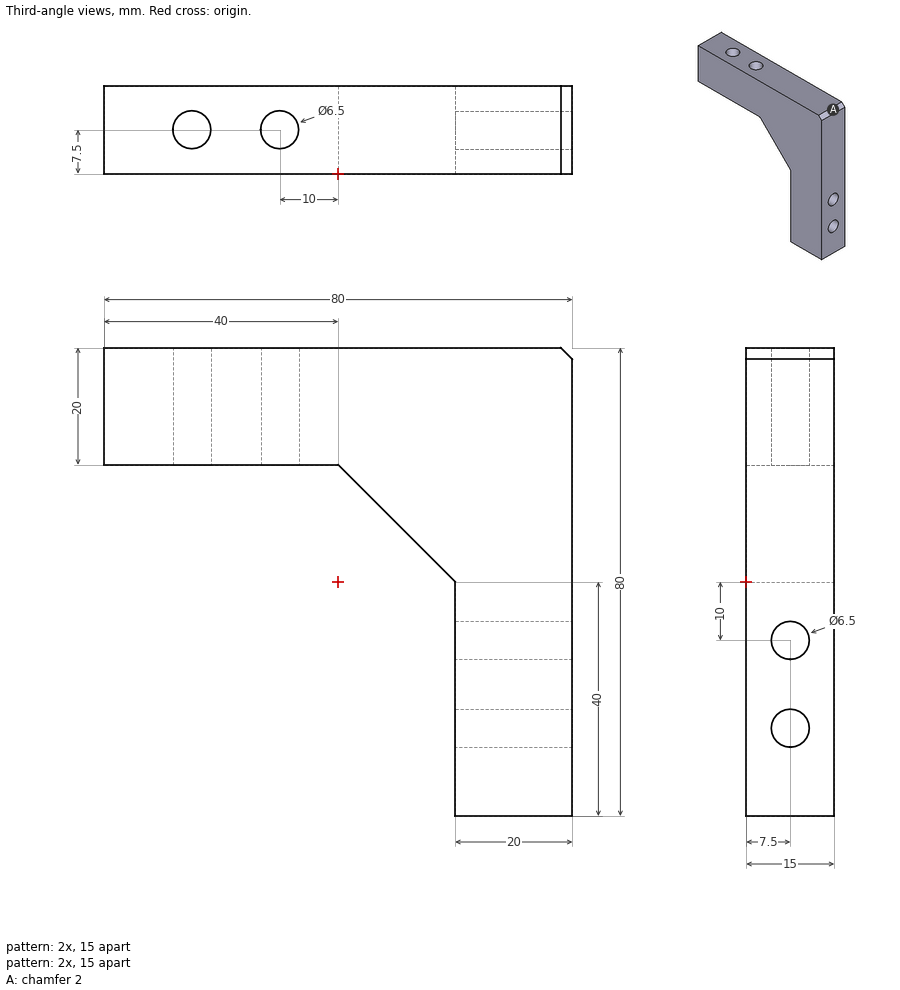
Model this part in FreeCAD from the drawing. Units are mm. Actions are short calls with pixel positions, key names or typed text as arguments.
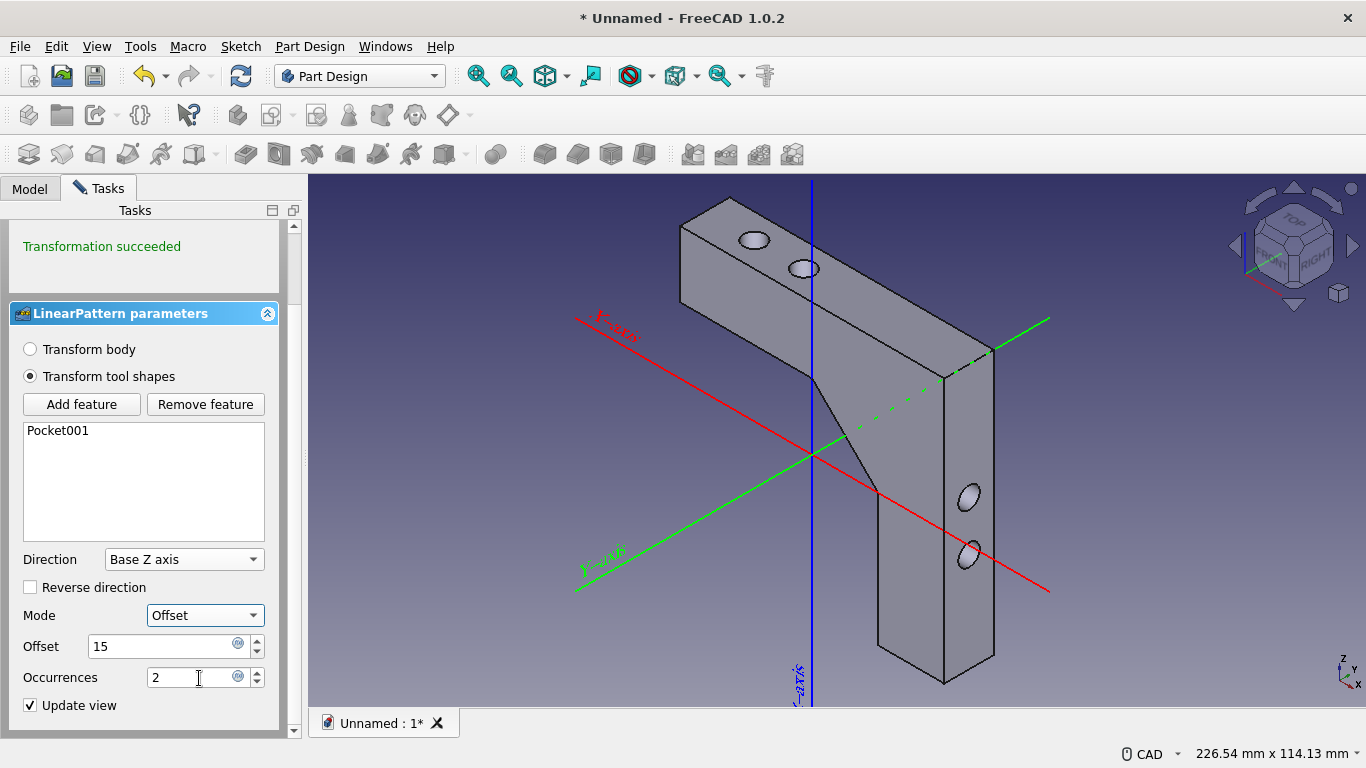
click(31, 587)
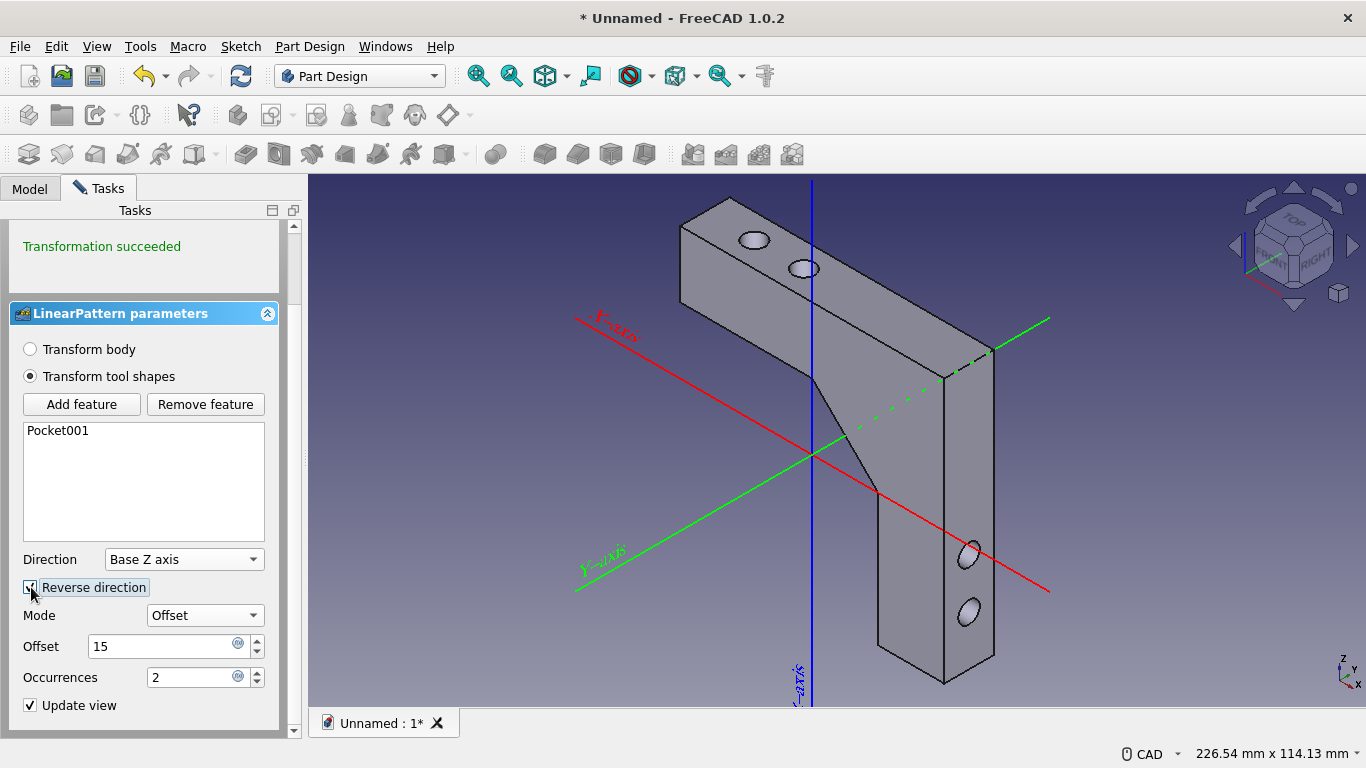
scroll(294, 479, up, 3)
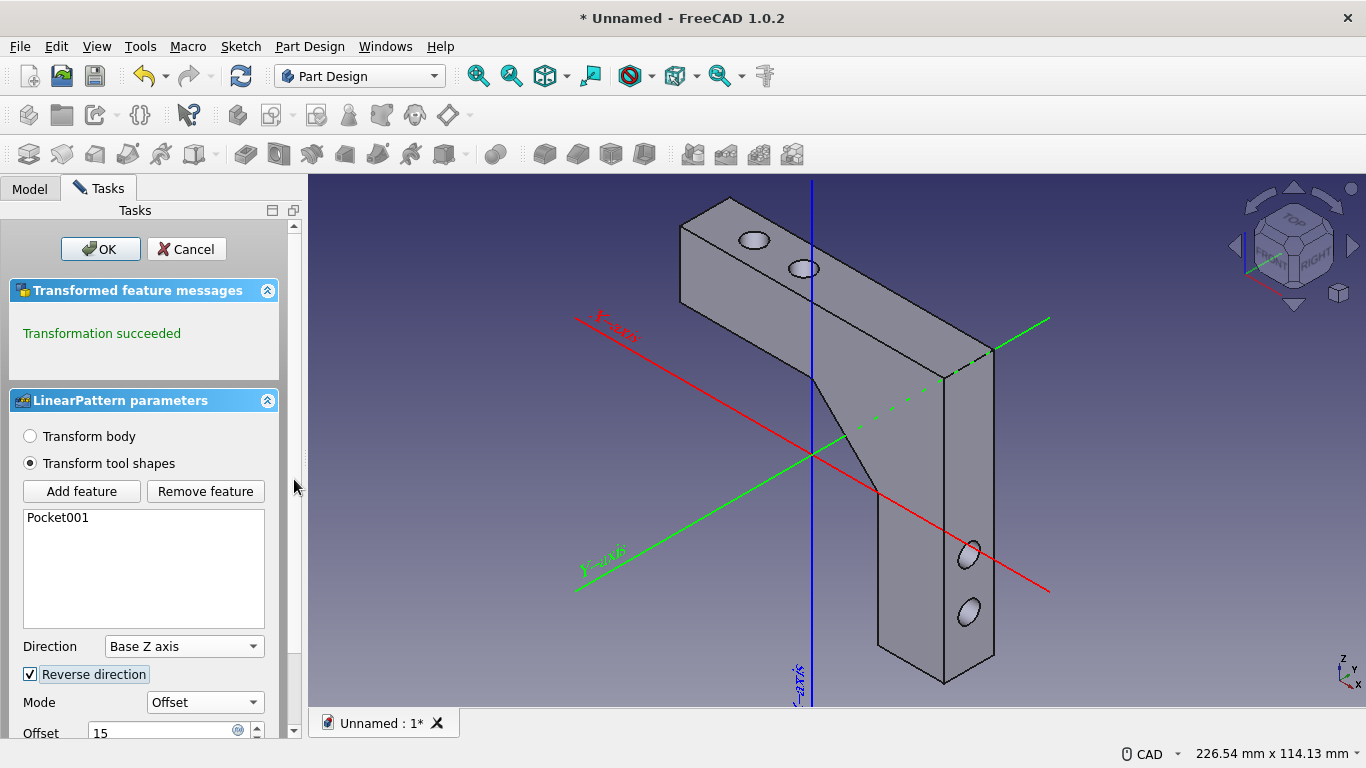
click(101, 249)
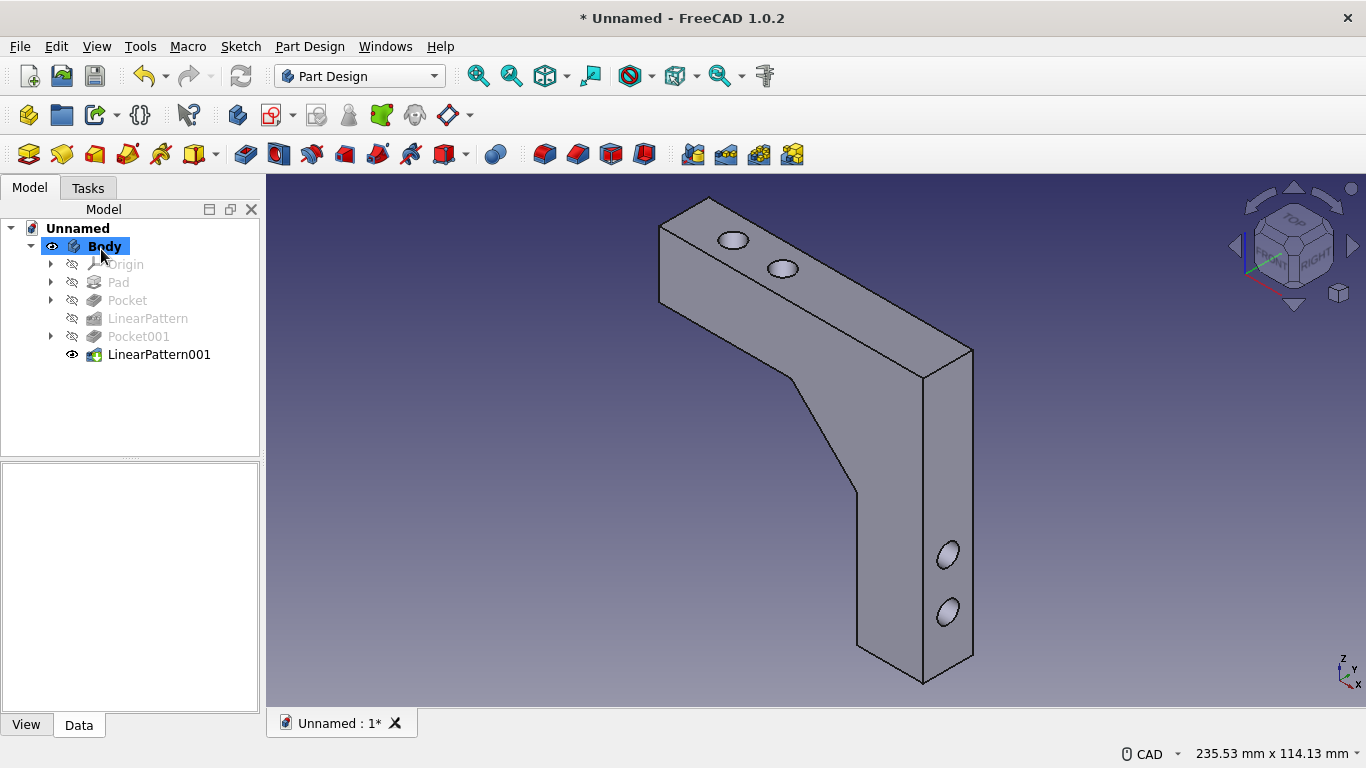
click(948, 363)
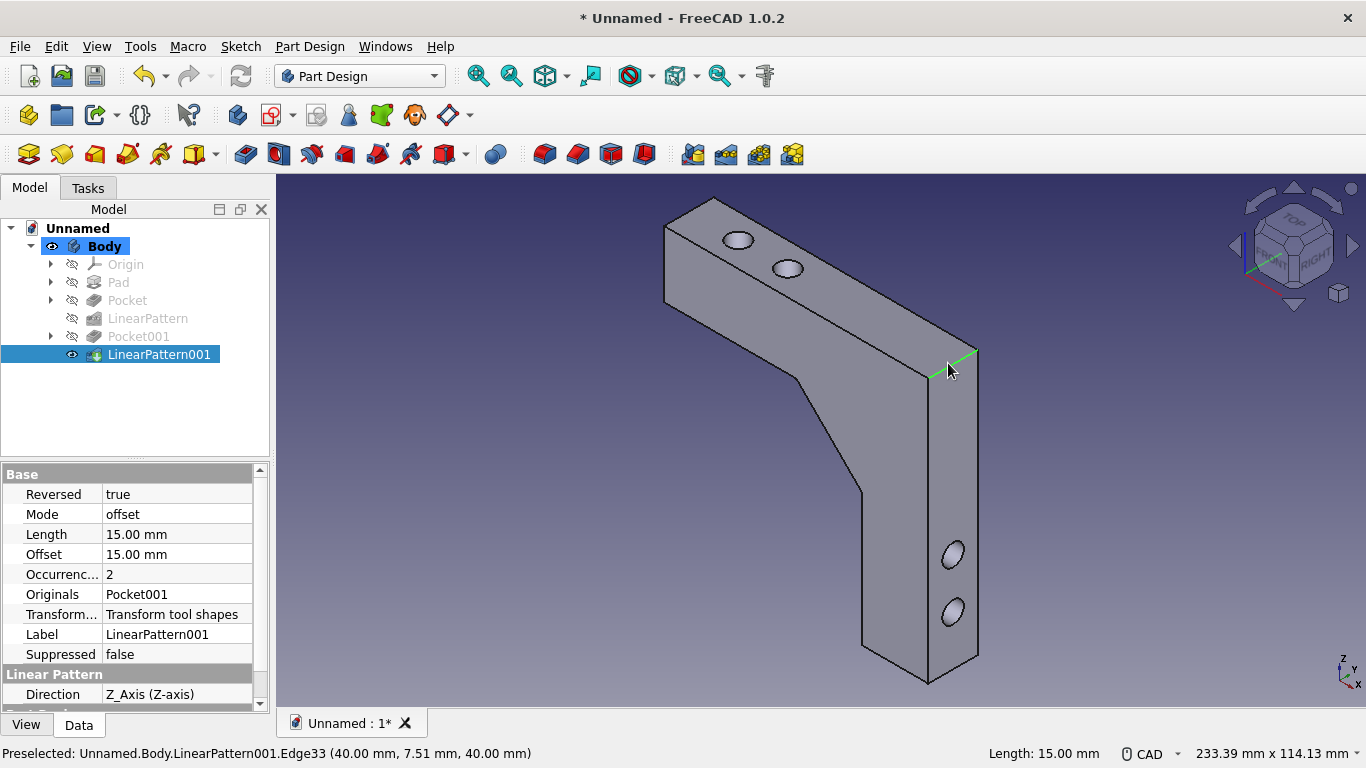
click(578, 154)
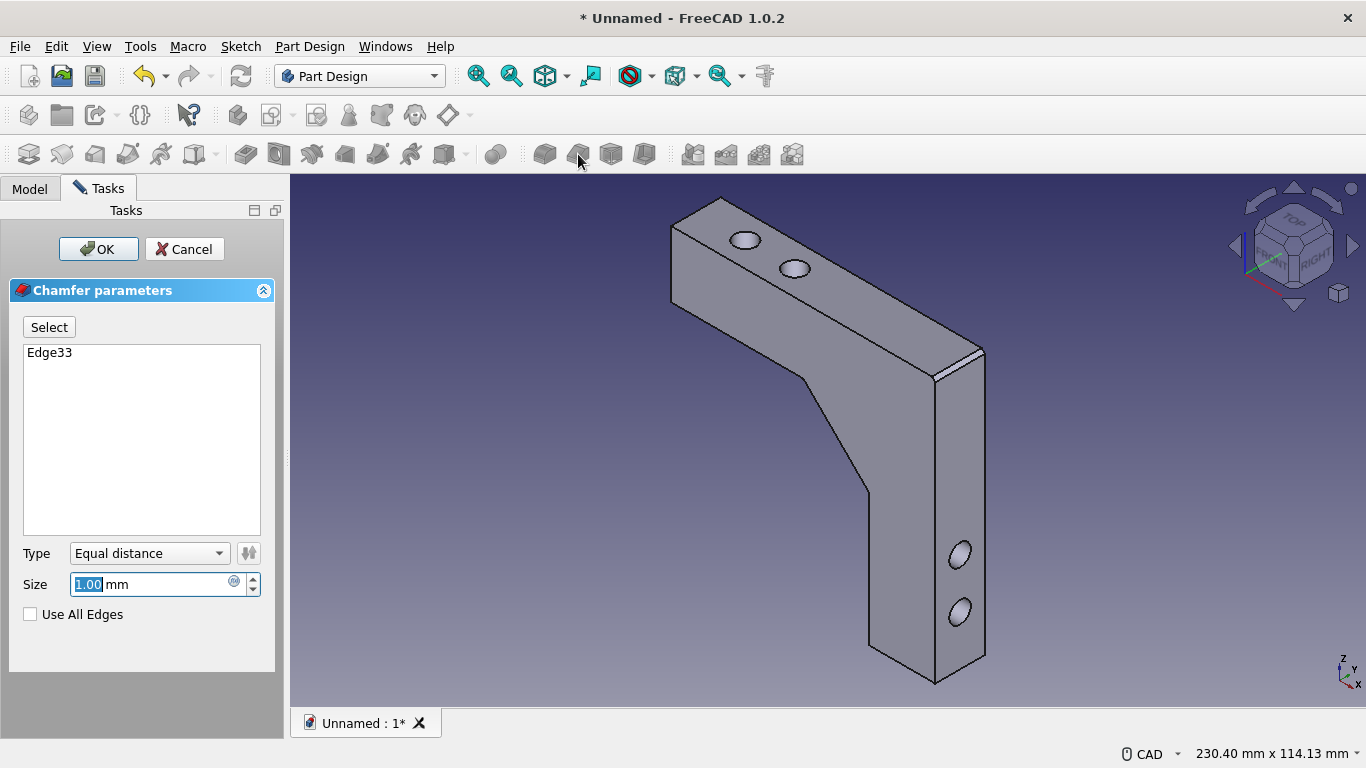
text(2)
key(Tab)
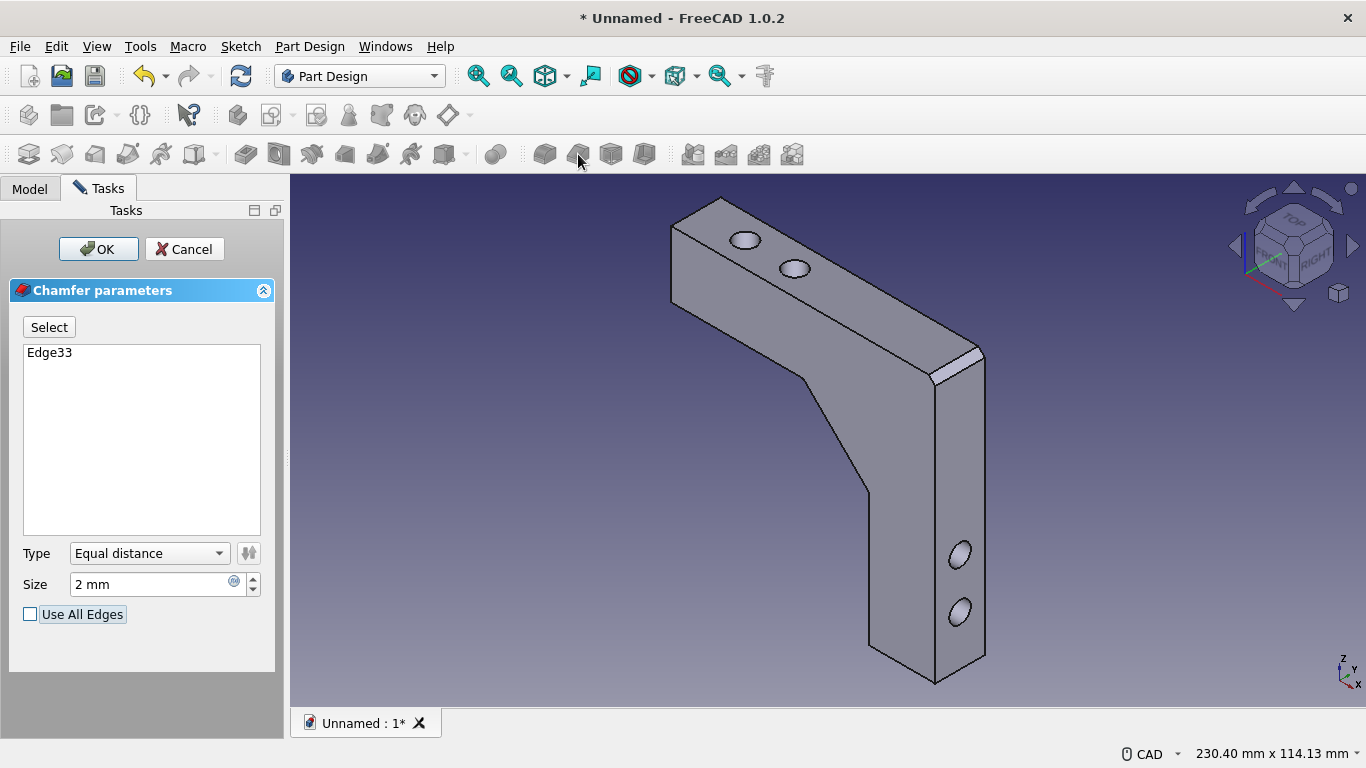
click(99, 249)